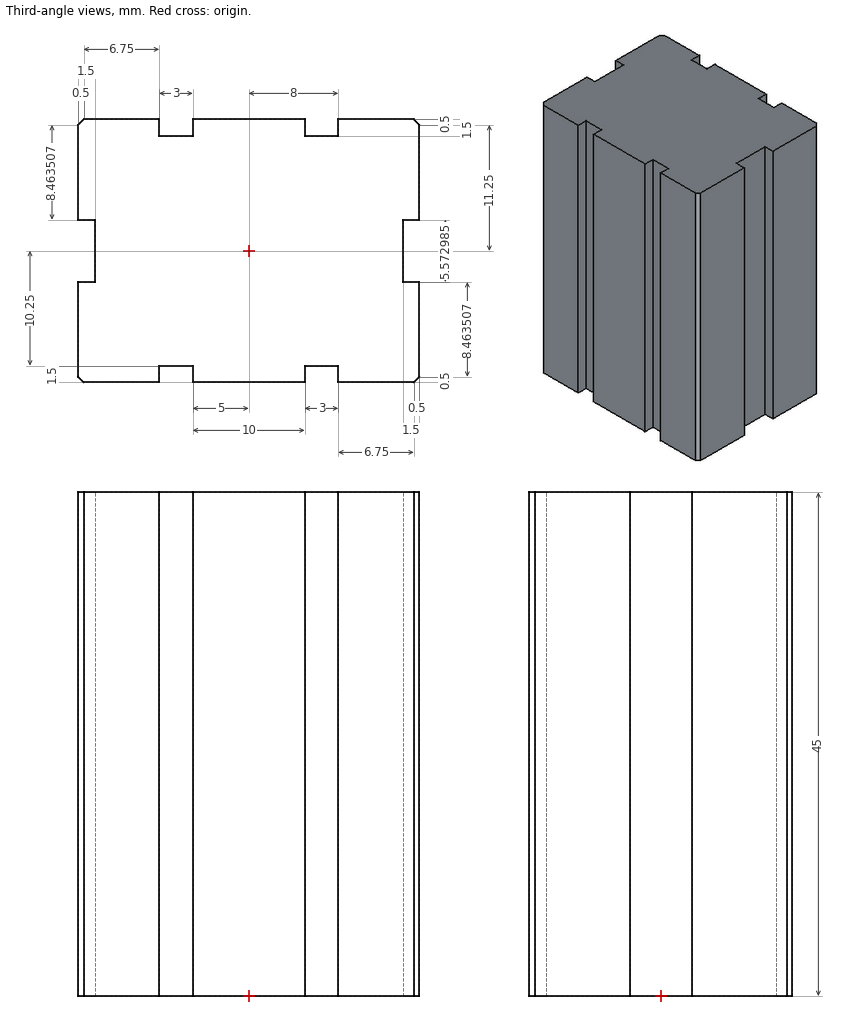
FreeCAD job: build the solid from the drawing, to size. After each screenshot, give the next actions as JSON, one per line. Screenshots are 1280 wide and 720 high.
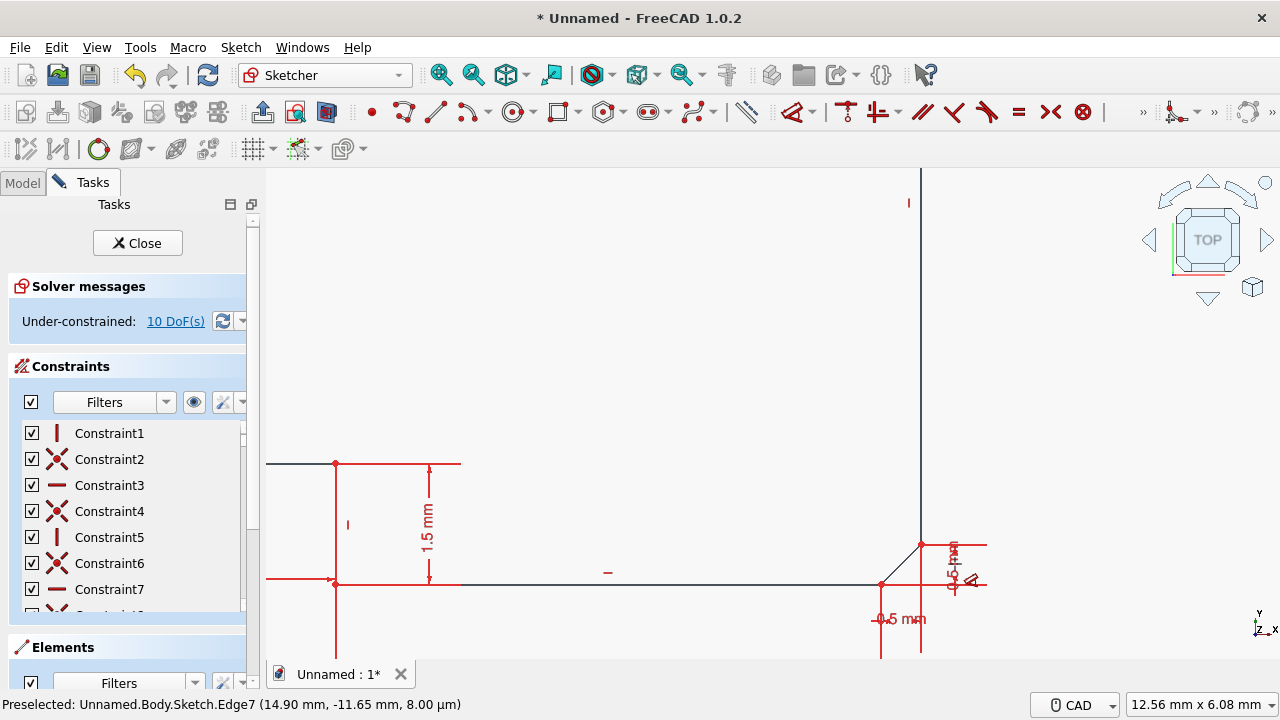
{"action": "scroll", "coordinate": [905, 568], "scroll_direction": "down", "scroll_amount": 9}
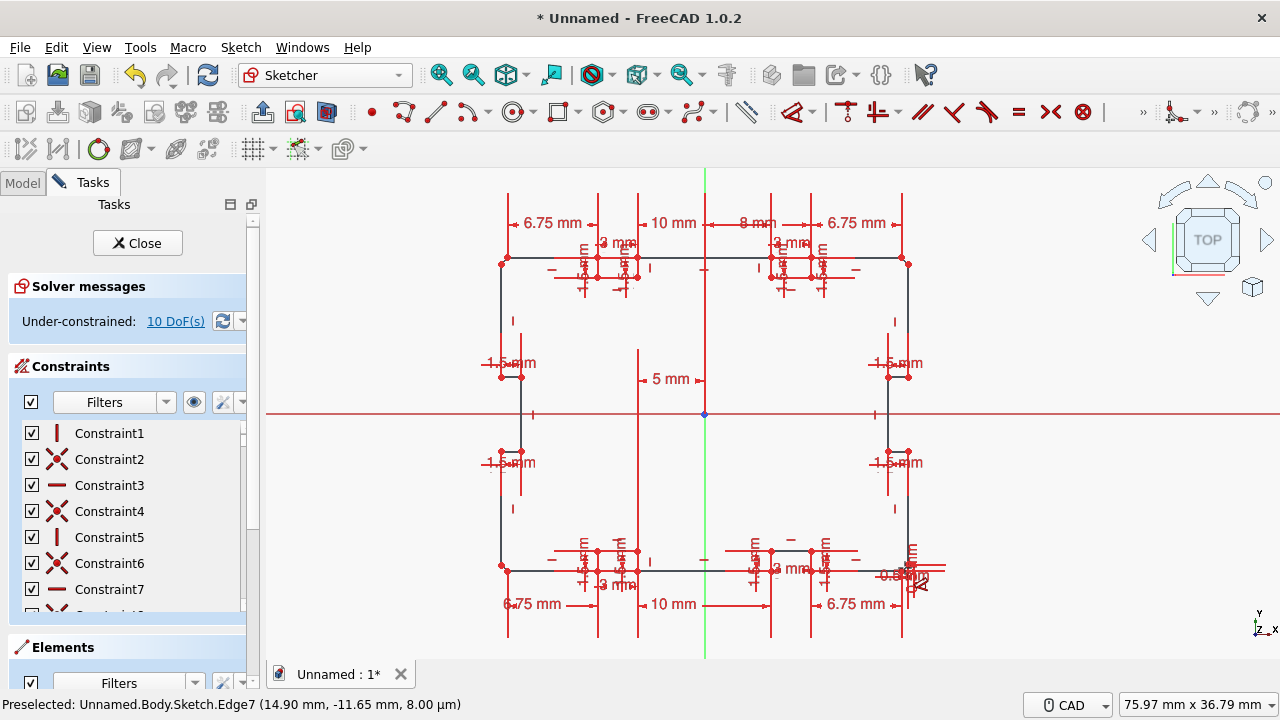
{"action": "scroll", "coordinate": [906, 263], "scroll_direction": "up", "scroll_amount": 9}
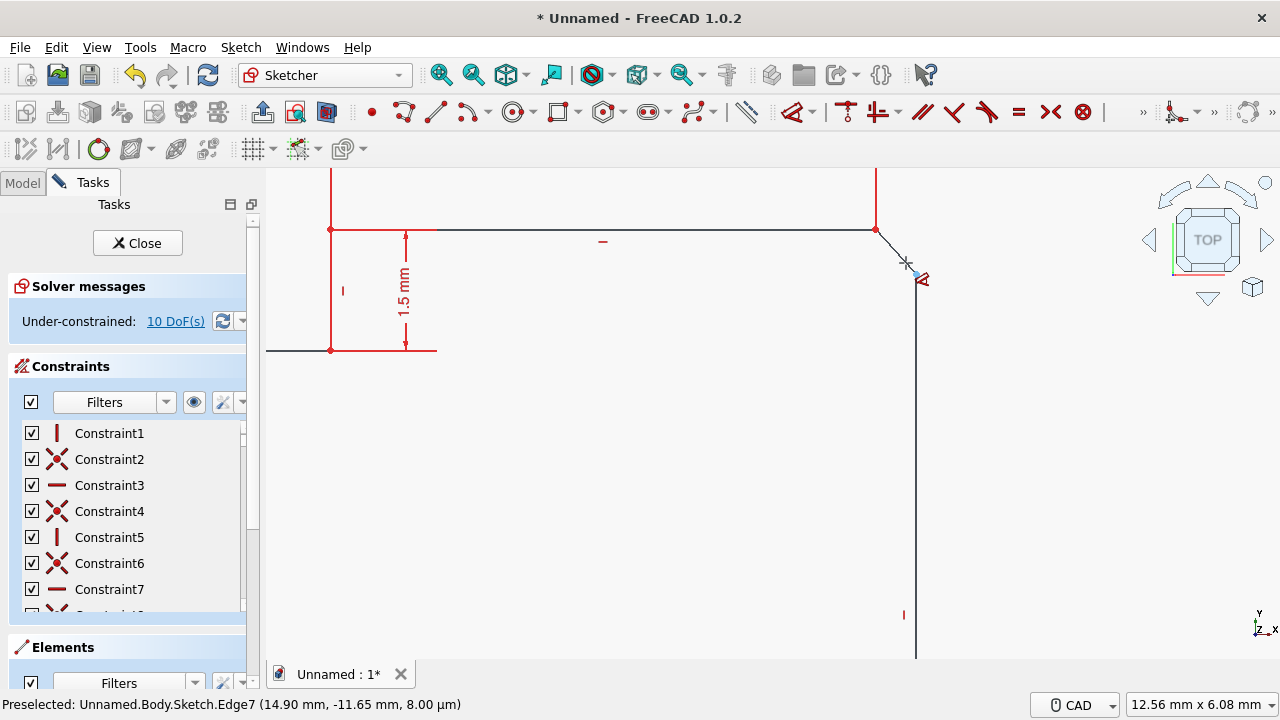
{"action": "left_click", "coordinate": [904, 261]}
{"action": "left_click", "coordinate": [950, 252]}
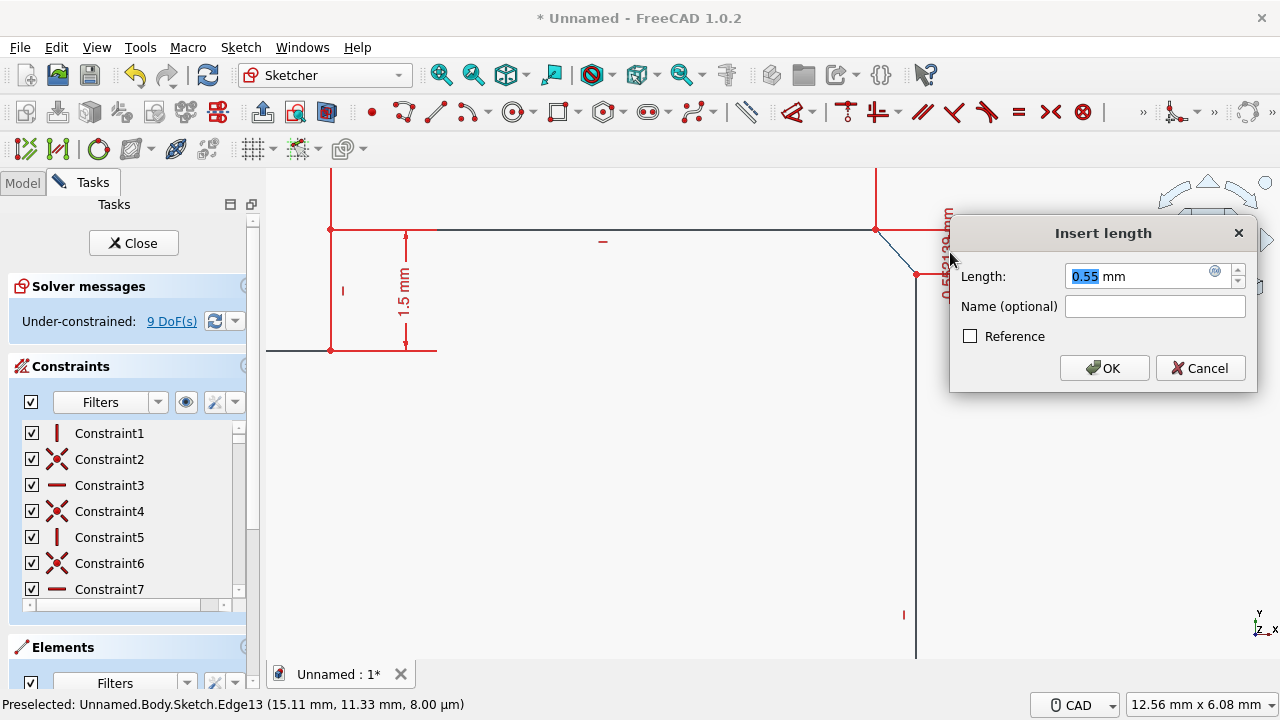
{"action": "type", "text": "0.5"}
{"action": "key", "text": "Return"}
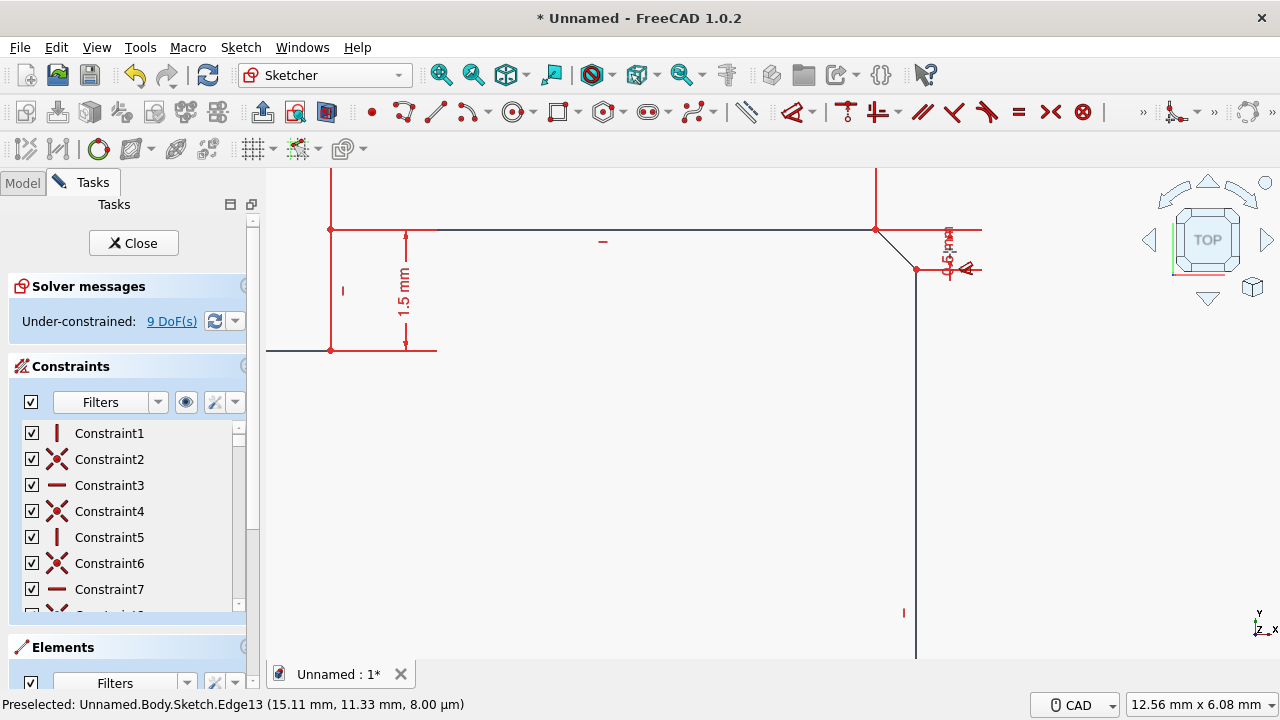
{"action": "scroll", "coordinate": [906, 263], "scroll_direction": "down", "scroll_amount": 9}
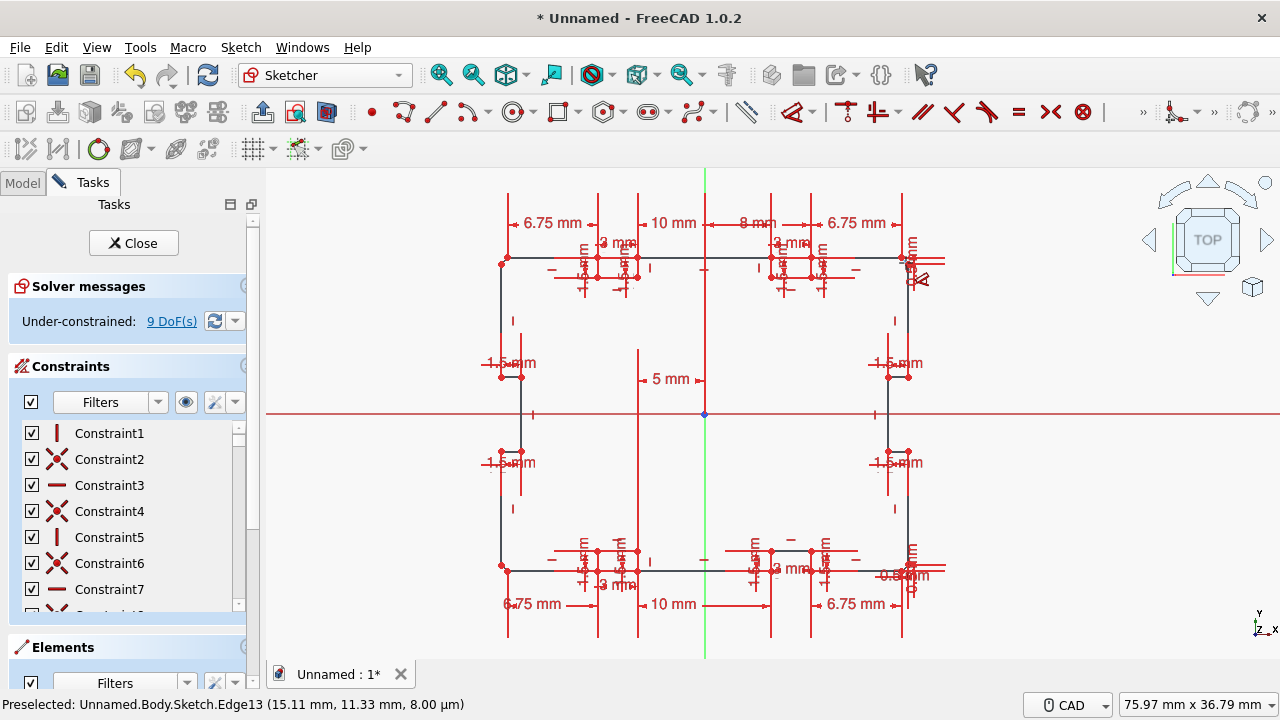
{"action": "scroll", "coordinate": [506, 260], "scroll_direction": "up", "scroll_amount": 9}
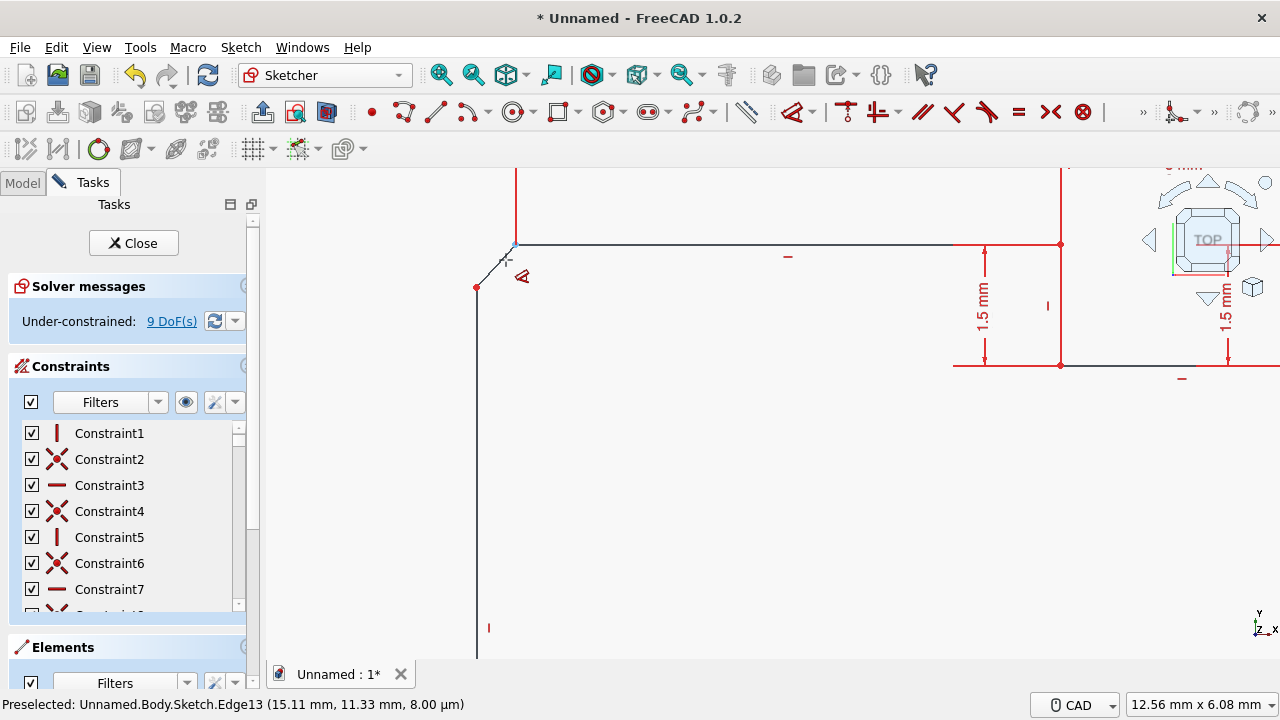
{"action": "left_click", "coordinate": [504, 257]}
{"action": "left_click", "coordinate": [496, 211]}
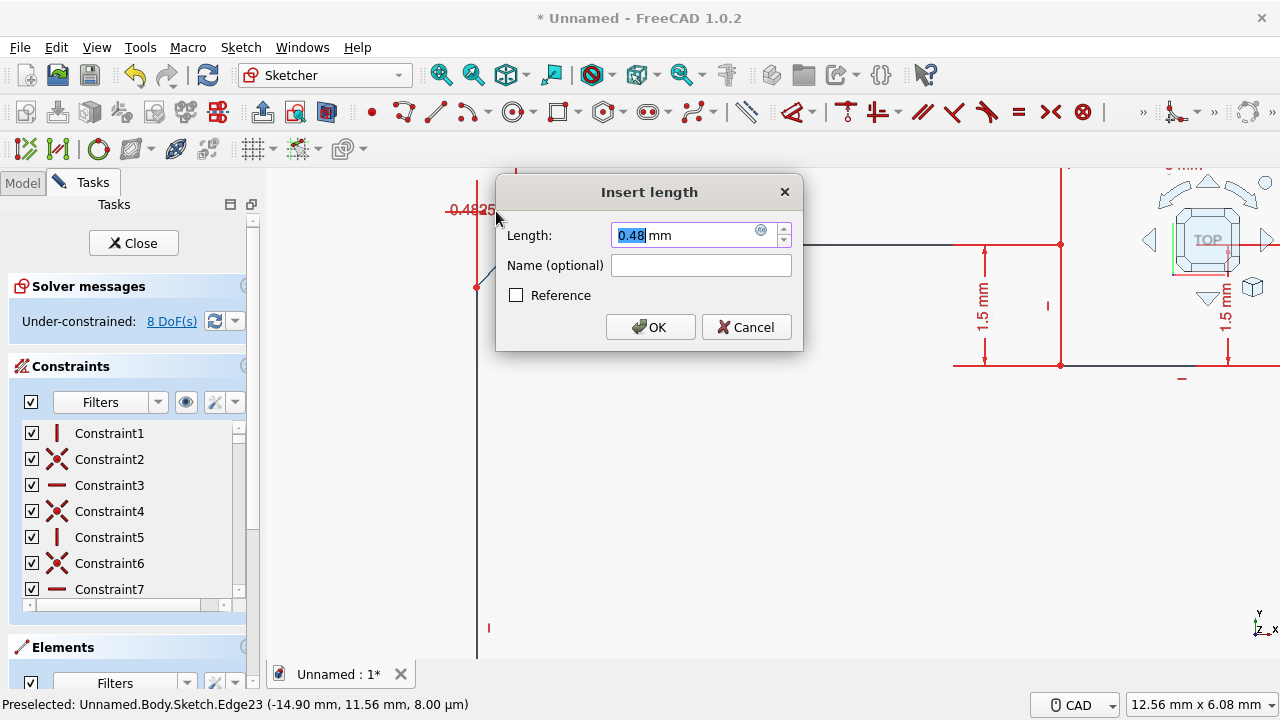
{"action": "type", "text": "0.5"}
{"action": "key", "text": "Return"}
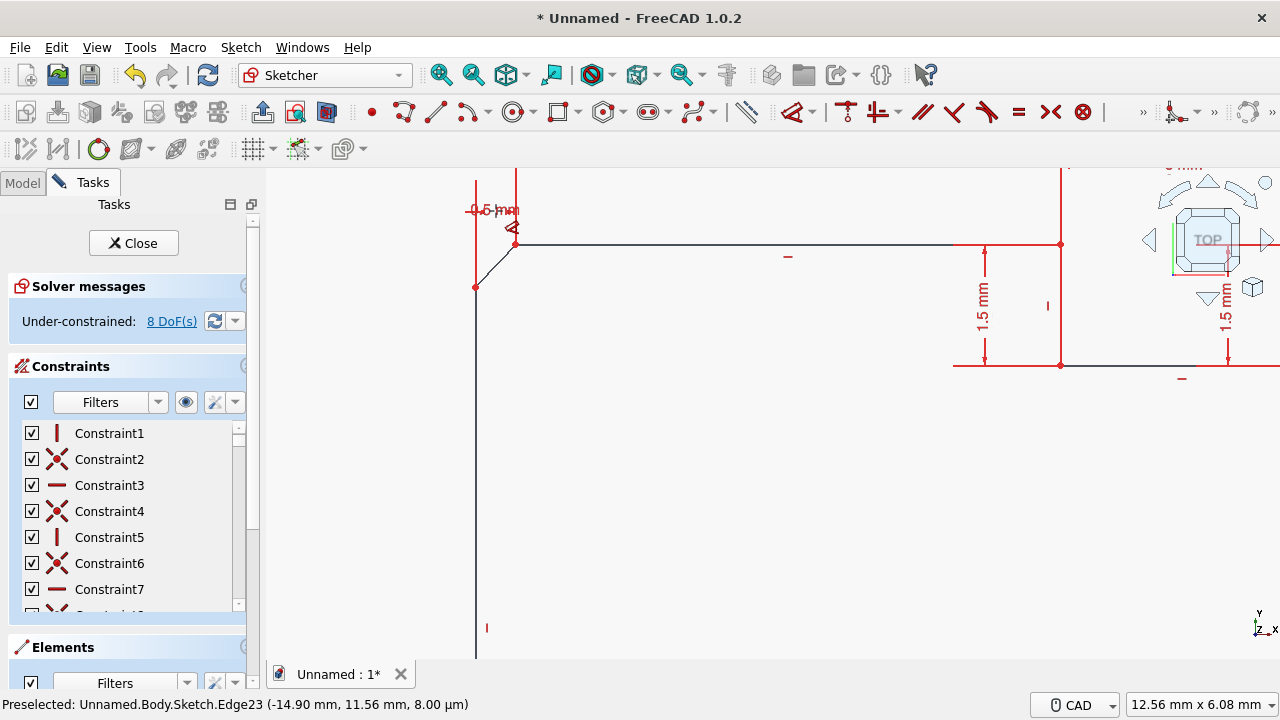
{"action": "left_click", "coordinate": [504, 257]}
{"action": "left_click", "coordinate": [442, 266]}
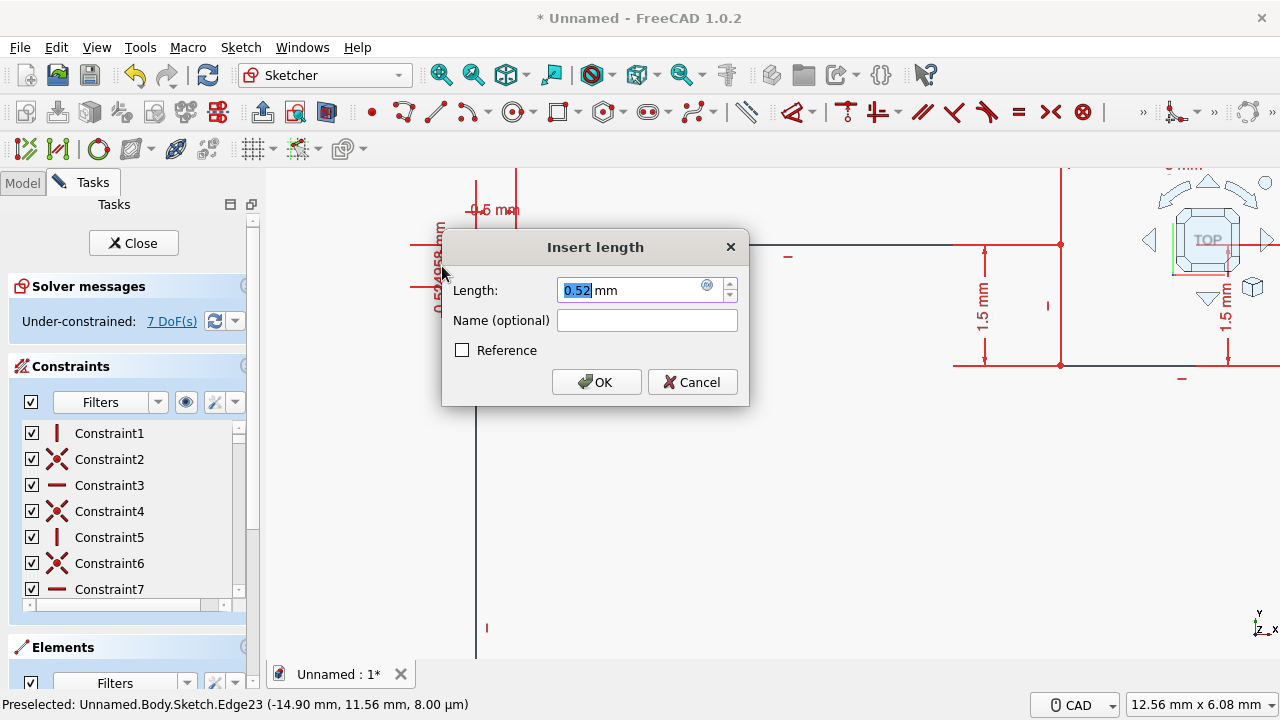
{"action": "type", "text": "0.5"}
{"action": "key", "text": "Return"}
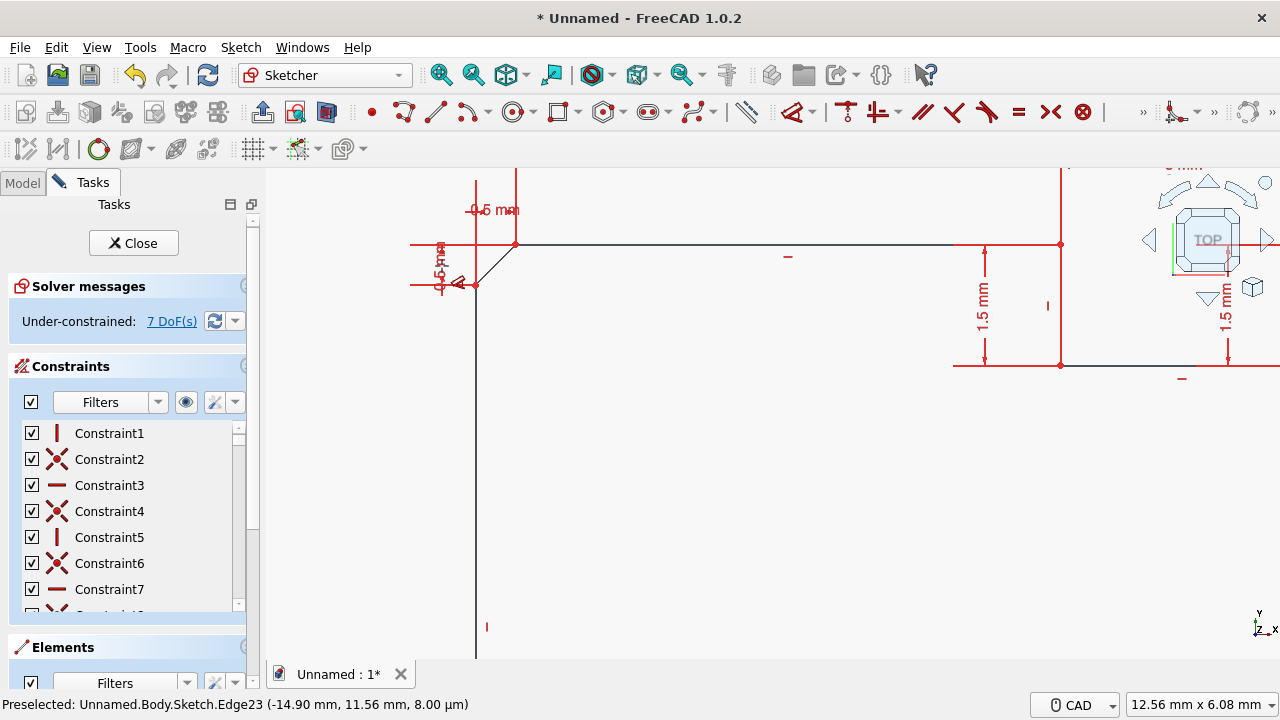
{"action": "scroll", "coordinate": [506, 260], "scroll_direction": "down", "scroll_amount": 9}